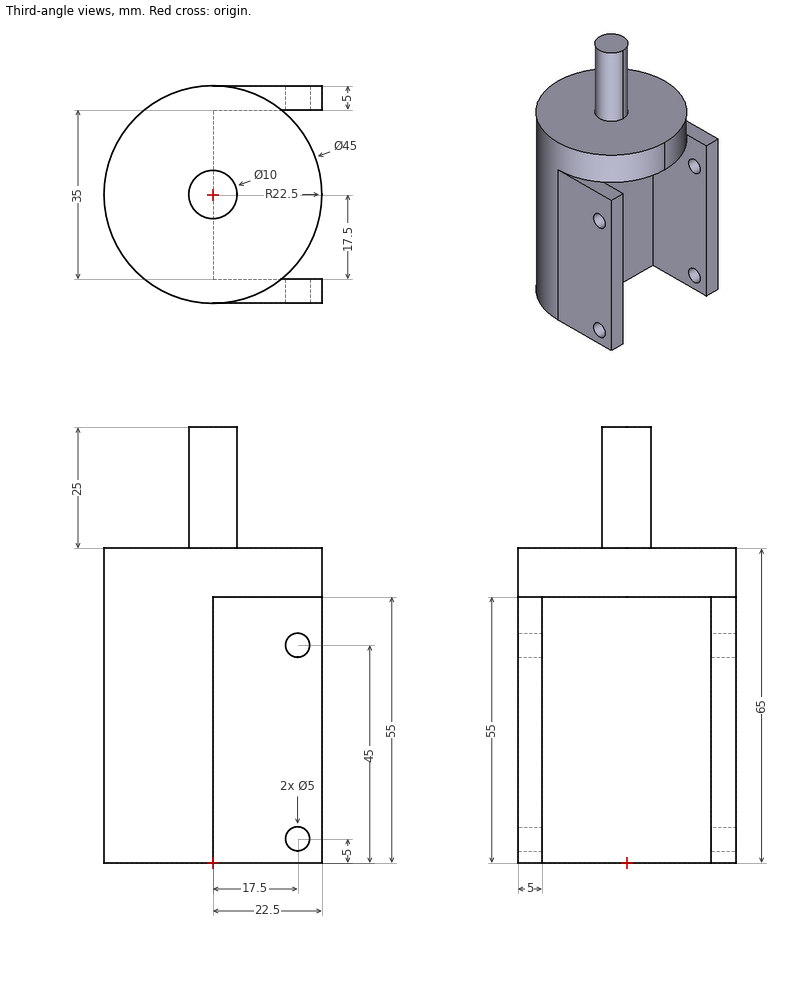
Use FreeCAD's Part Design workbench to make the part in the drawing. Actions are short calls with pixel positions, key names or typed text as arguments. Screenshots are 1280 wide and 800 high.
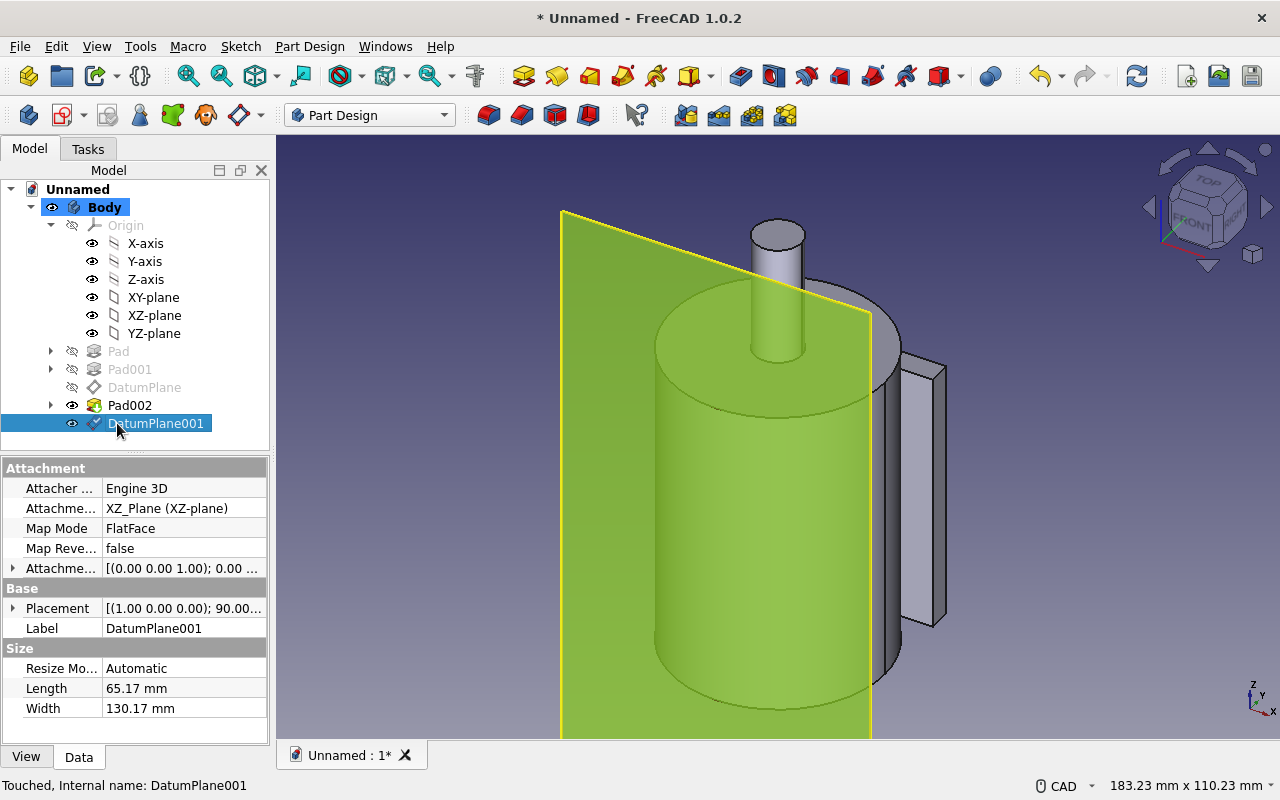
click(62, 116)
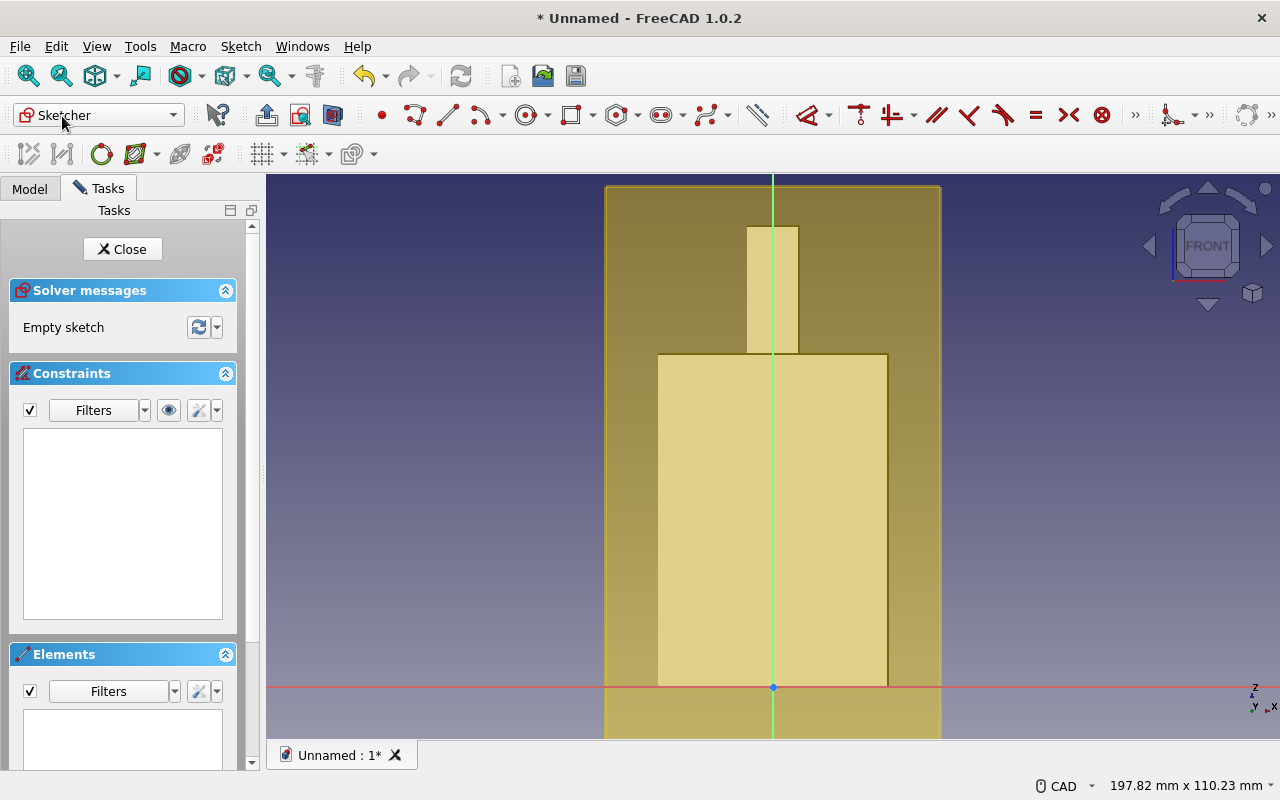
scroll(1115, 711, up, 1)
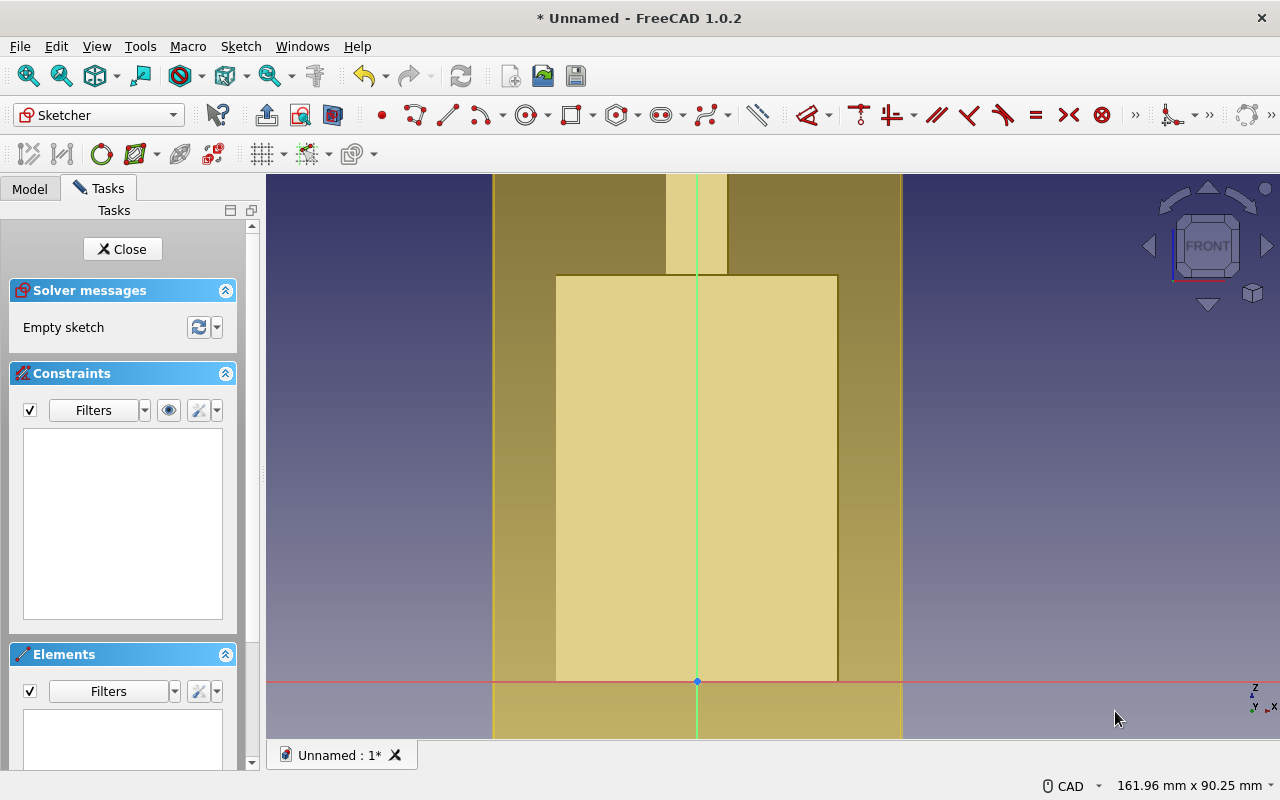
click(570, 116)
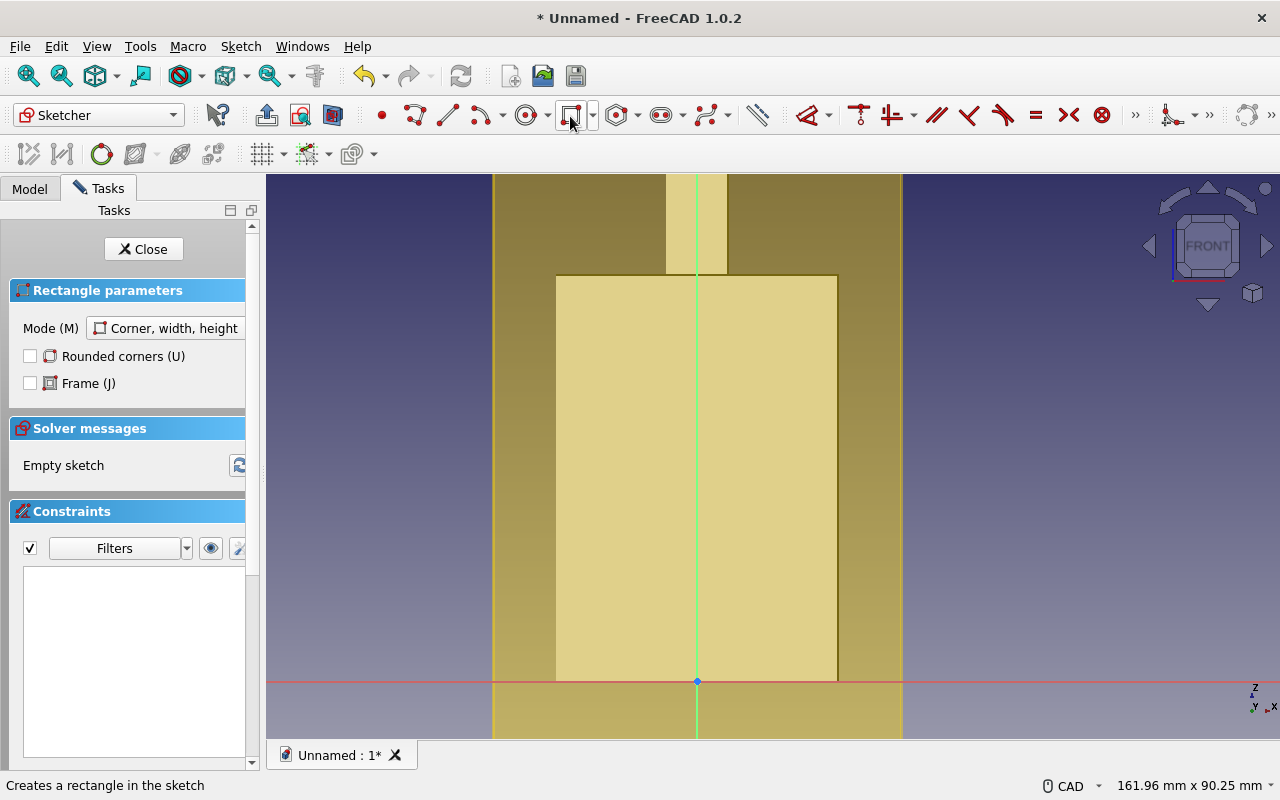
click(697, 682)
click(838, 337)
key(Escape)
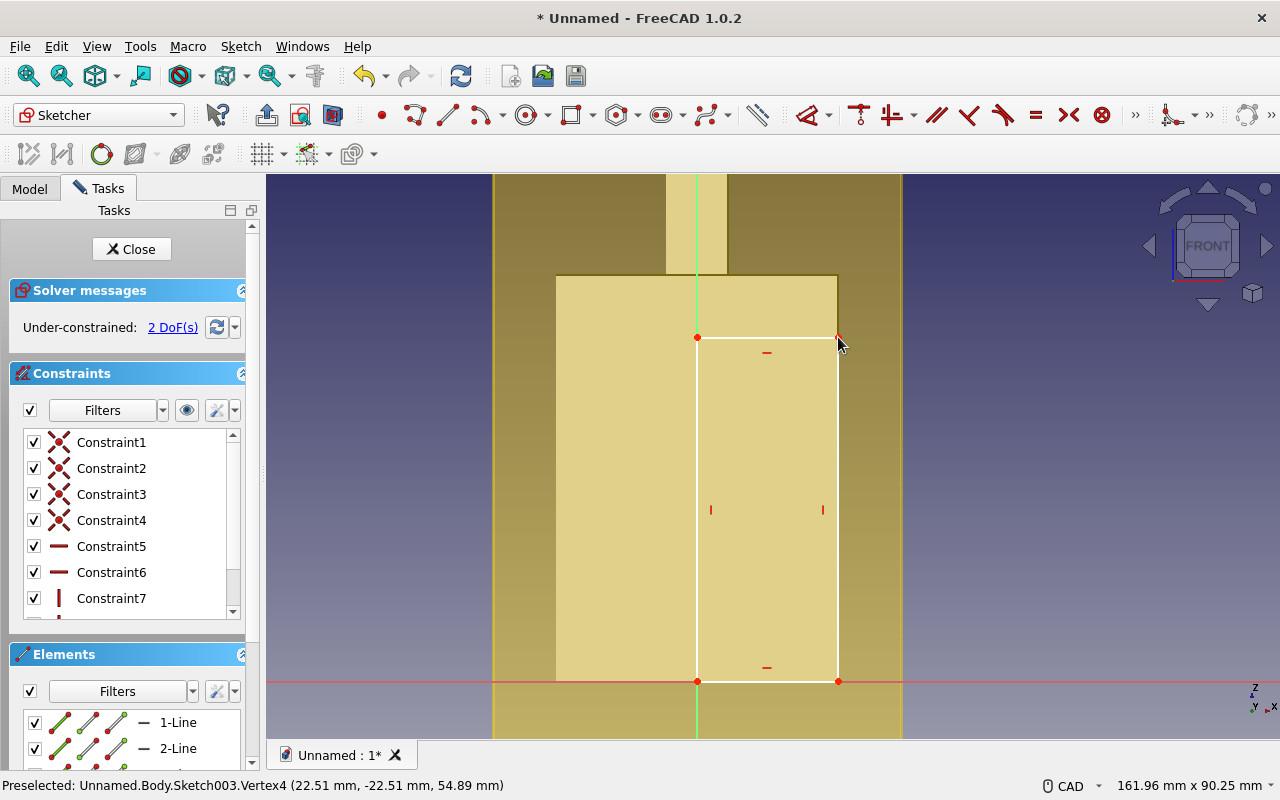
click(806, 116)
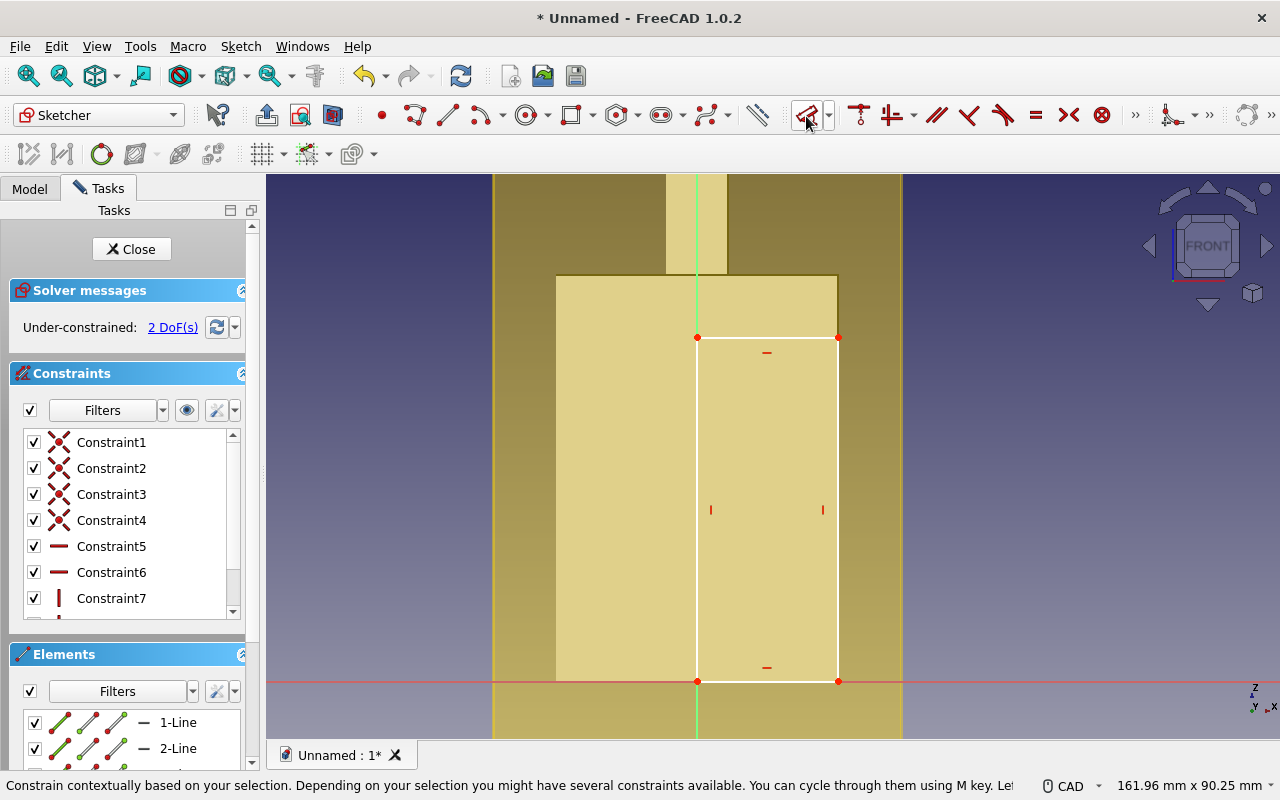
click(838, 579)
click(872, 510)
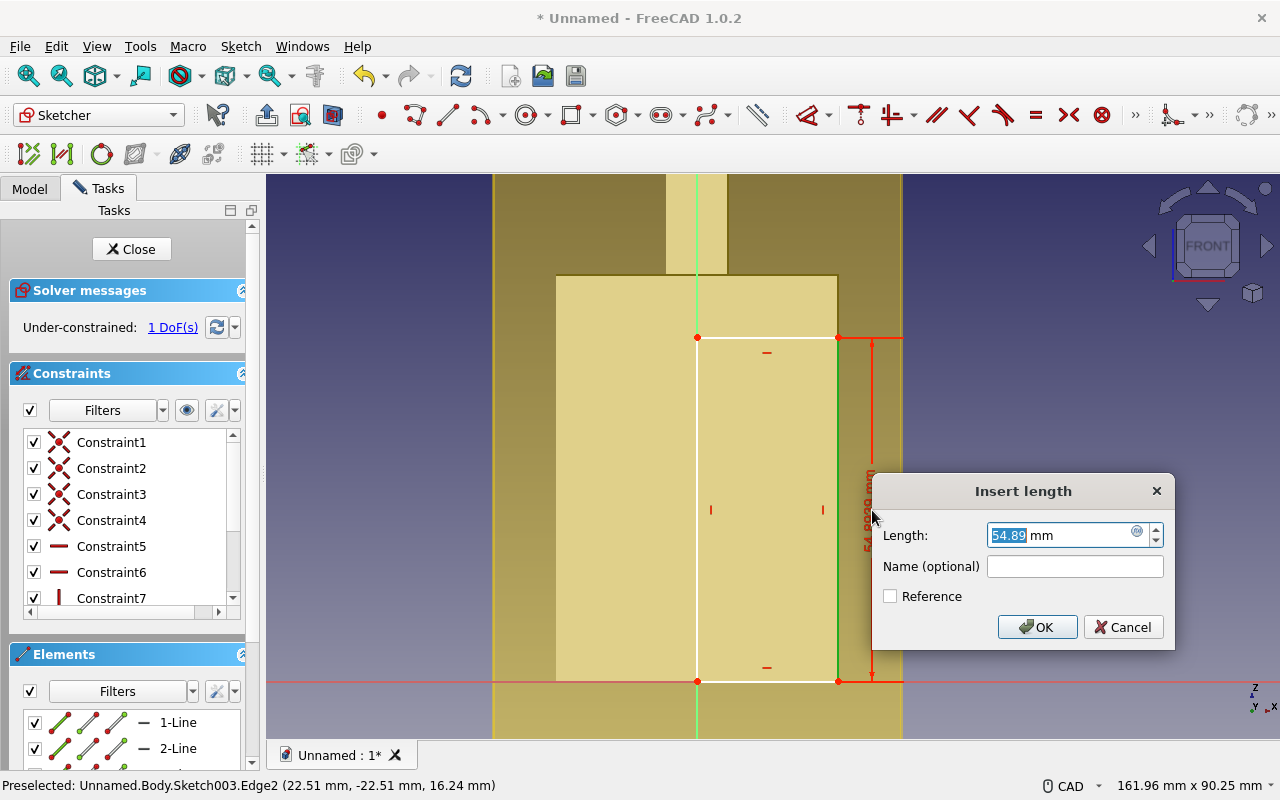
text(55)
key(Return)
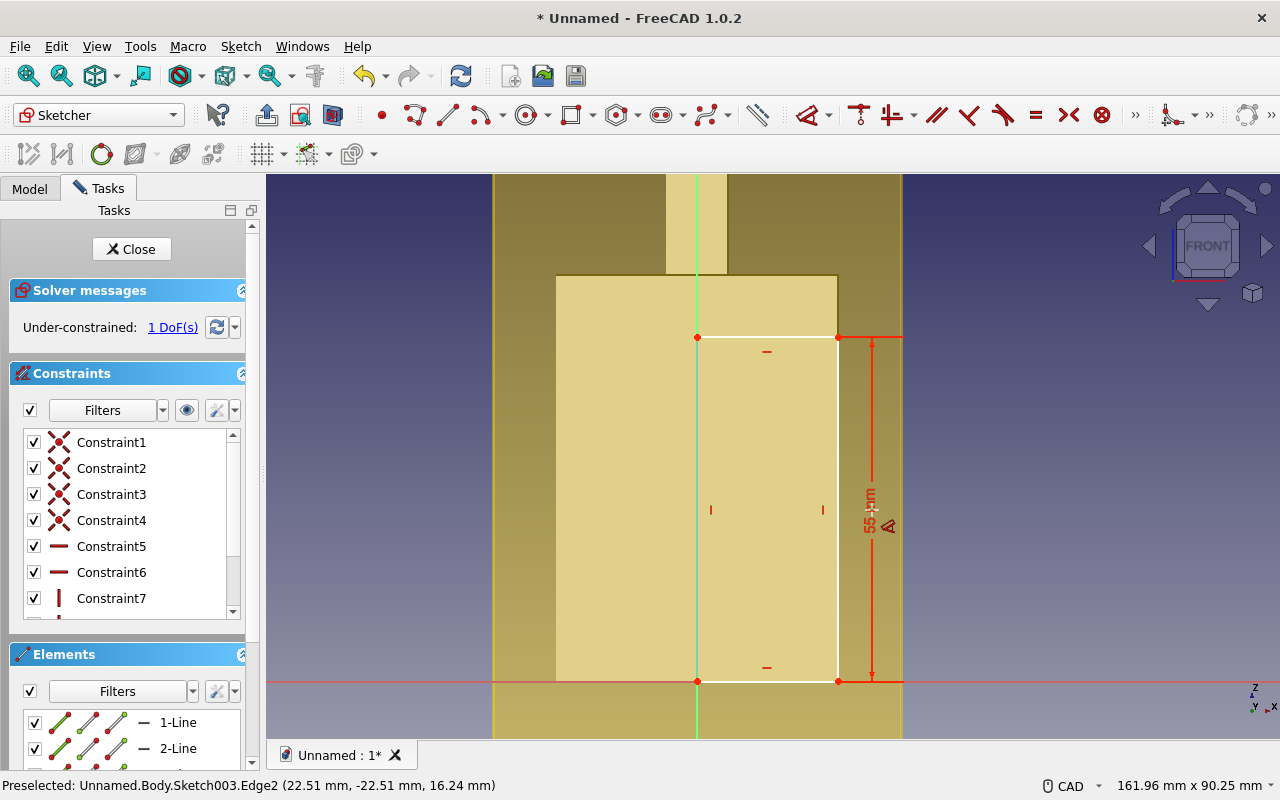
click(739, 682)
click(768, 648)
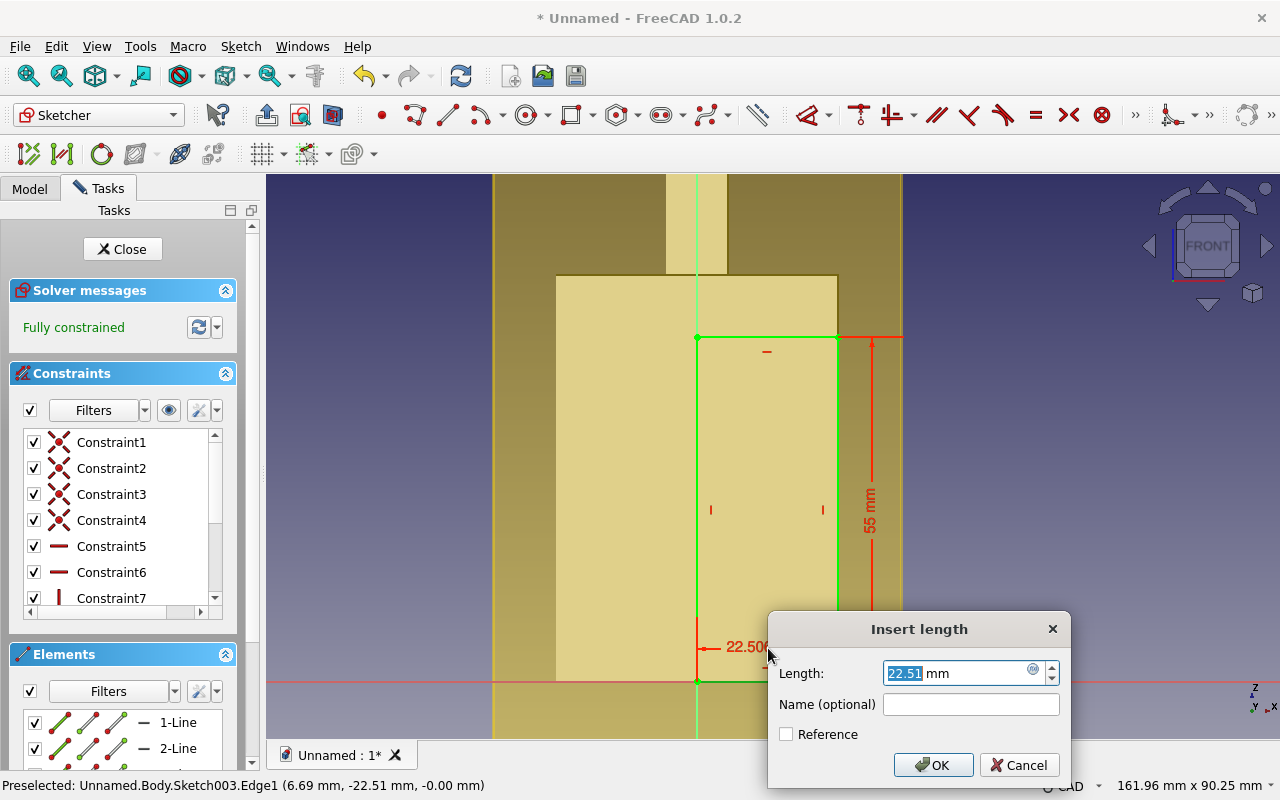
text(22.5)
key(Return)
key(Escape)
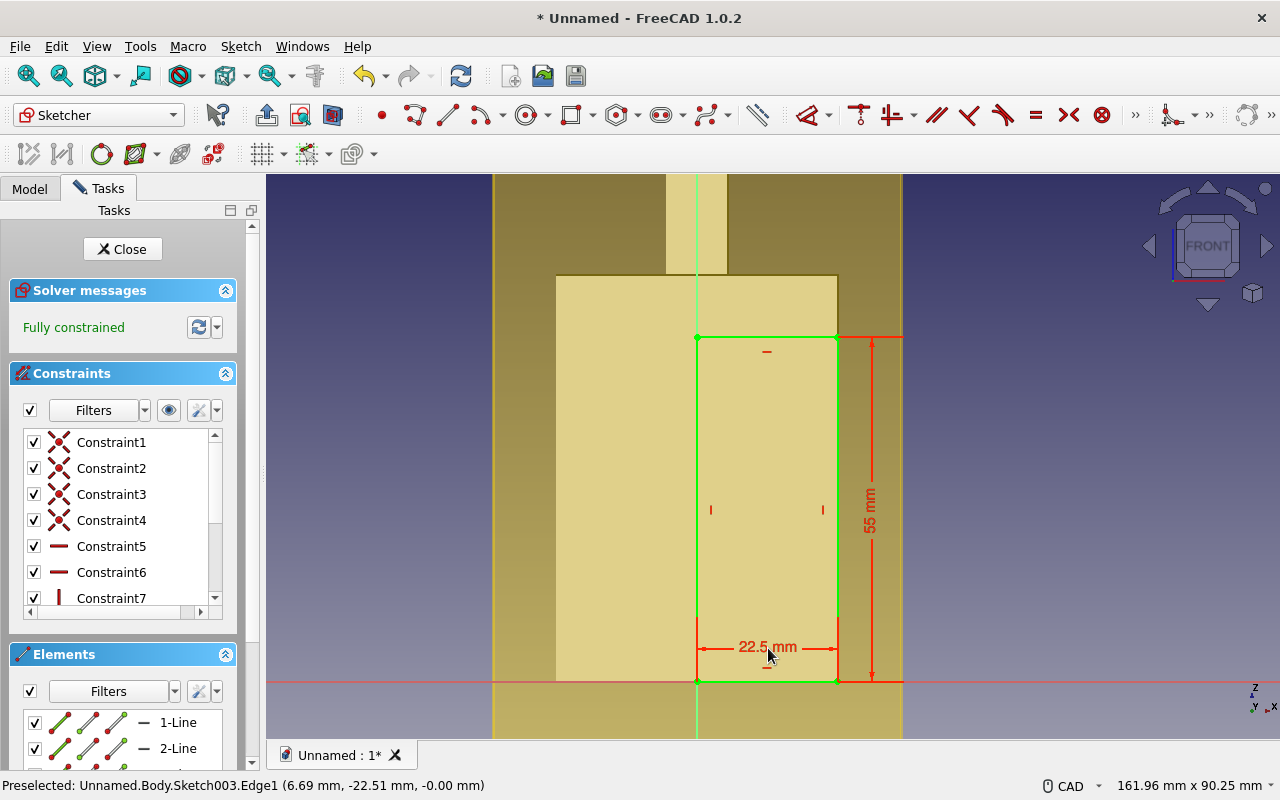
click(123, 249)